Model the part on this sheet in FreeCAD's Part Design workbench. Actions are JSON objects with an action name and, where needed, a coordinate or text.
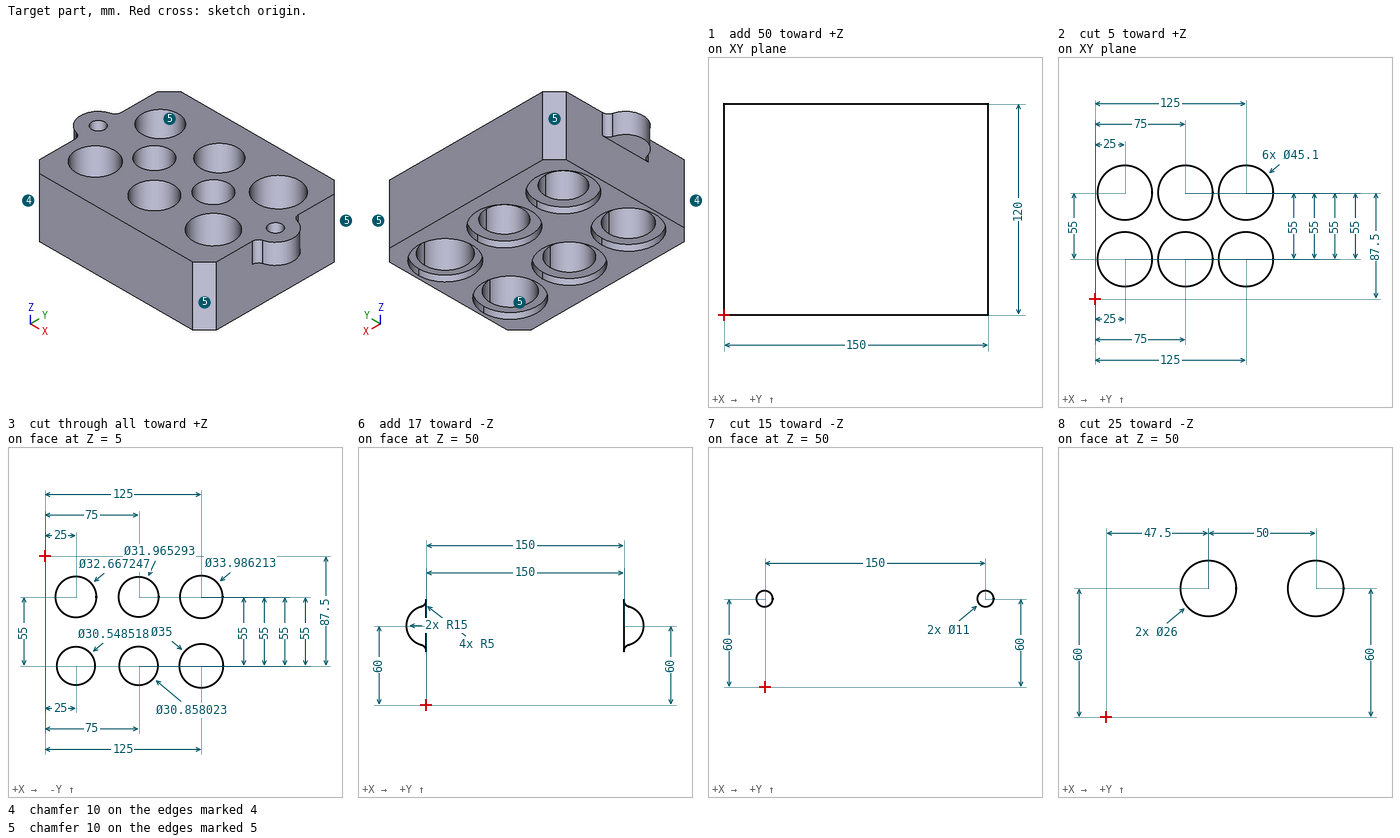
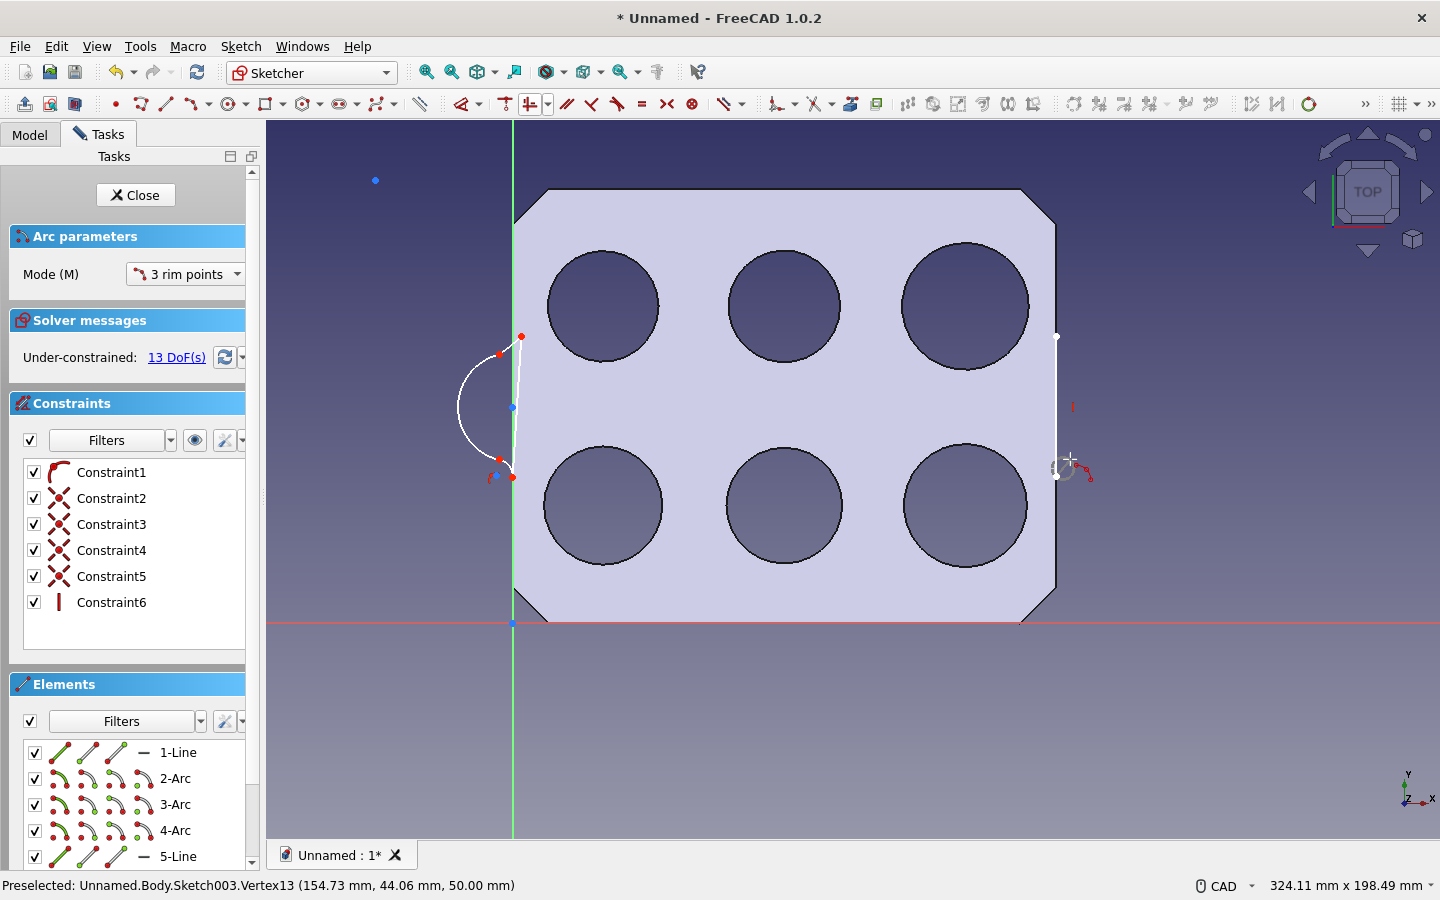
{"action": "scroll", "coordinate": [1060, 465], "scroll_direction": "up", "scroll_amount": 8}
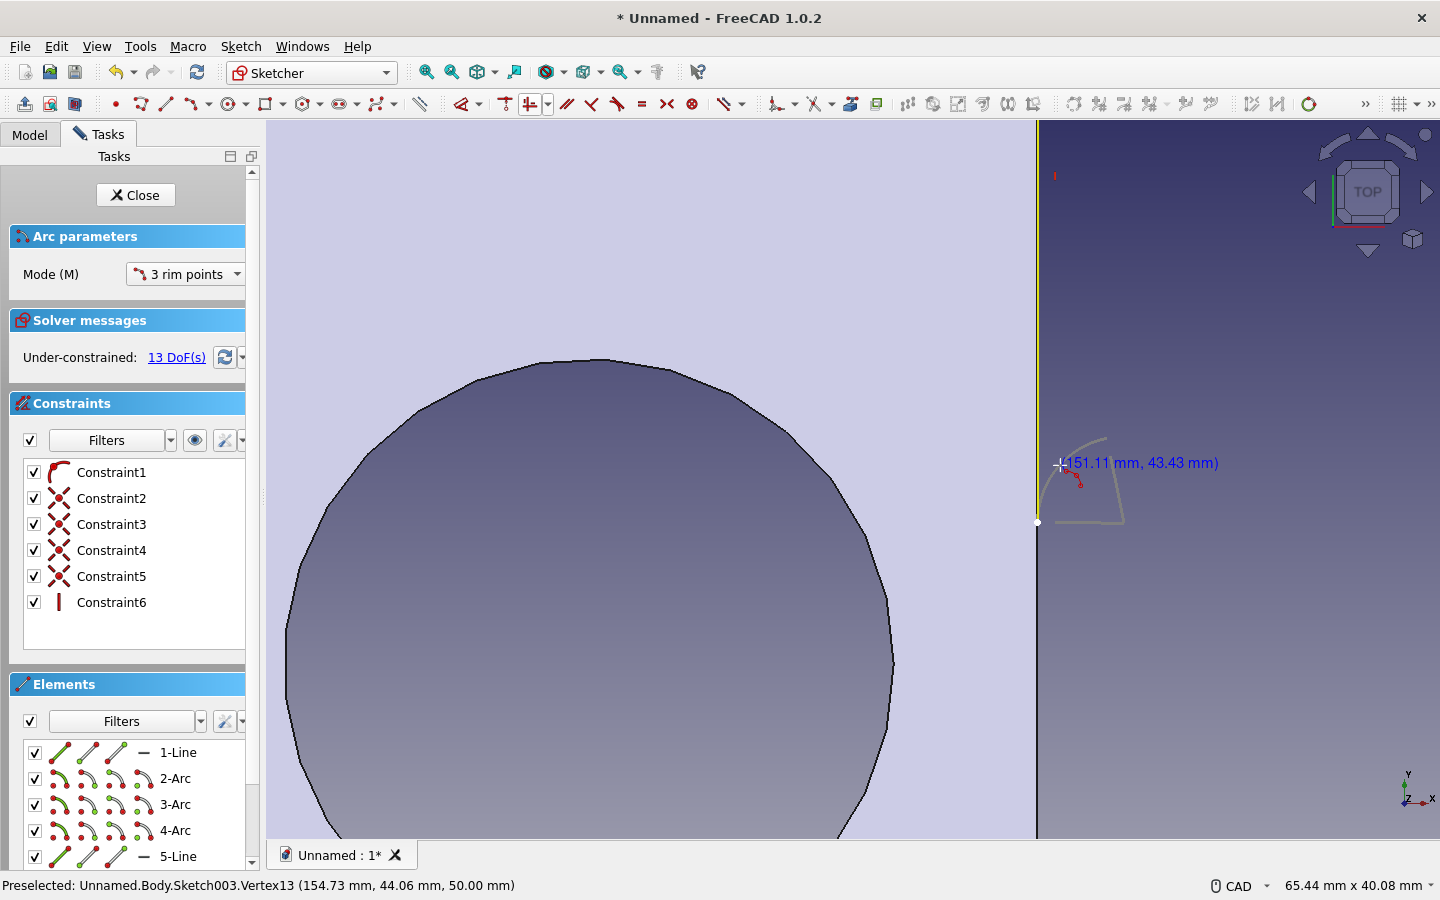
{"action": "left_click", "coordinate": [1056, 463]}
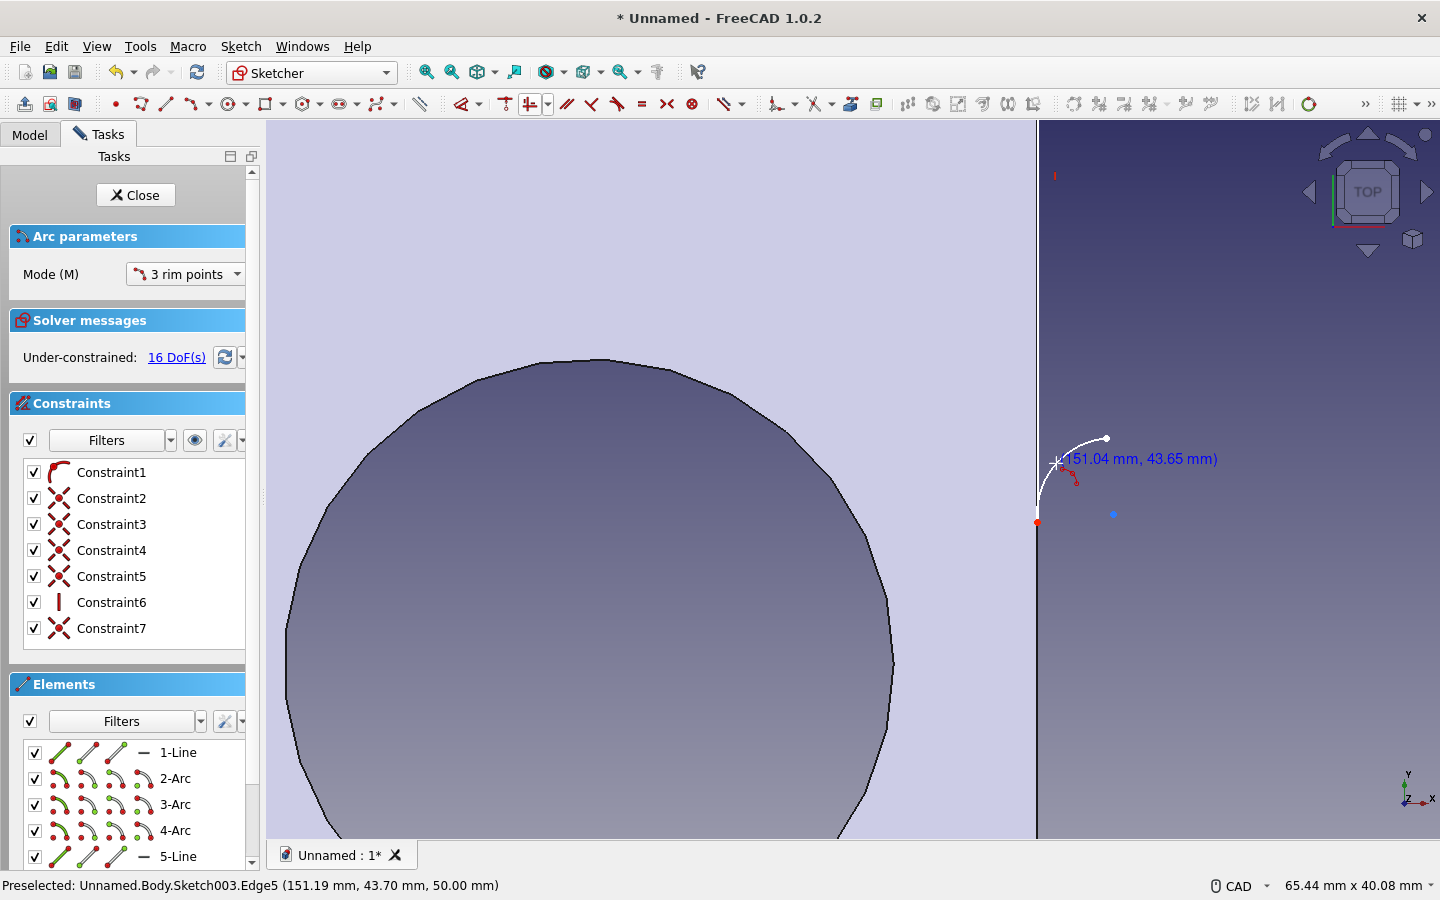
{"action": "scroll", "coordinate": [1061, 465], "scroll_direction": "down", "scroll_amount": 8}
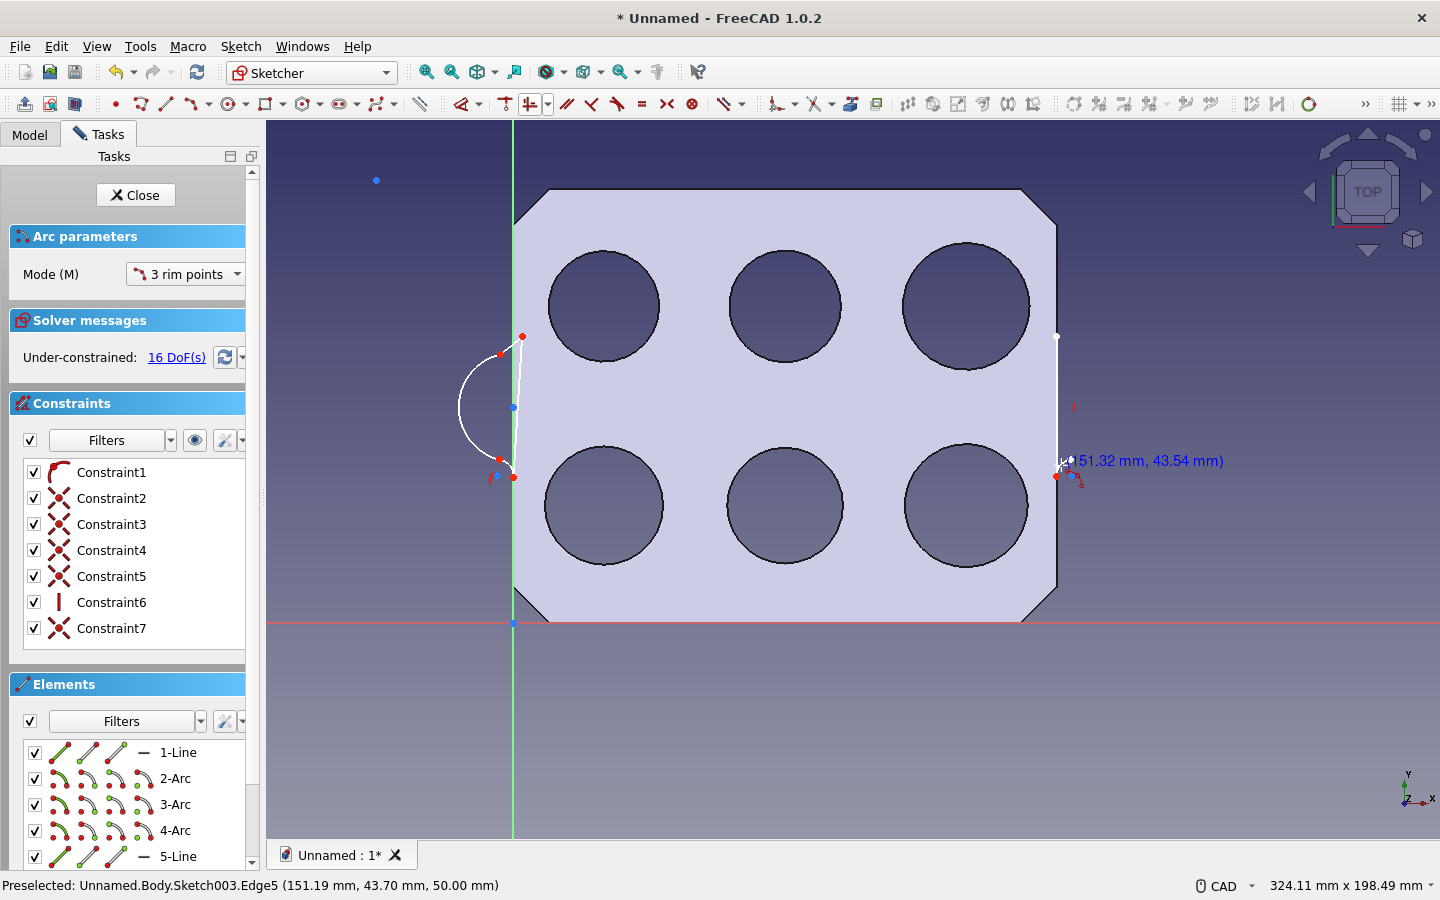
{"action": "left_click", "coordinate": [1071, 460]}
{"action": "left_click", "coordinate": [1070, 353]}
{"action": "left_click", "coordinate": [1111, 406]}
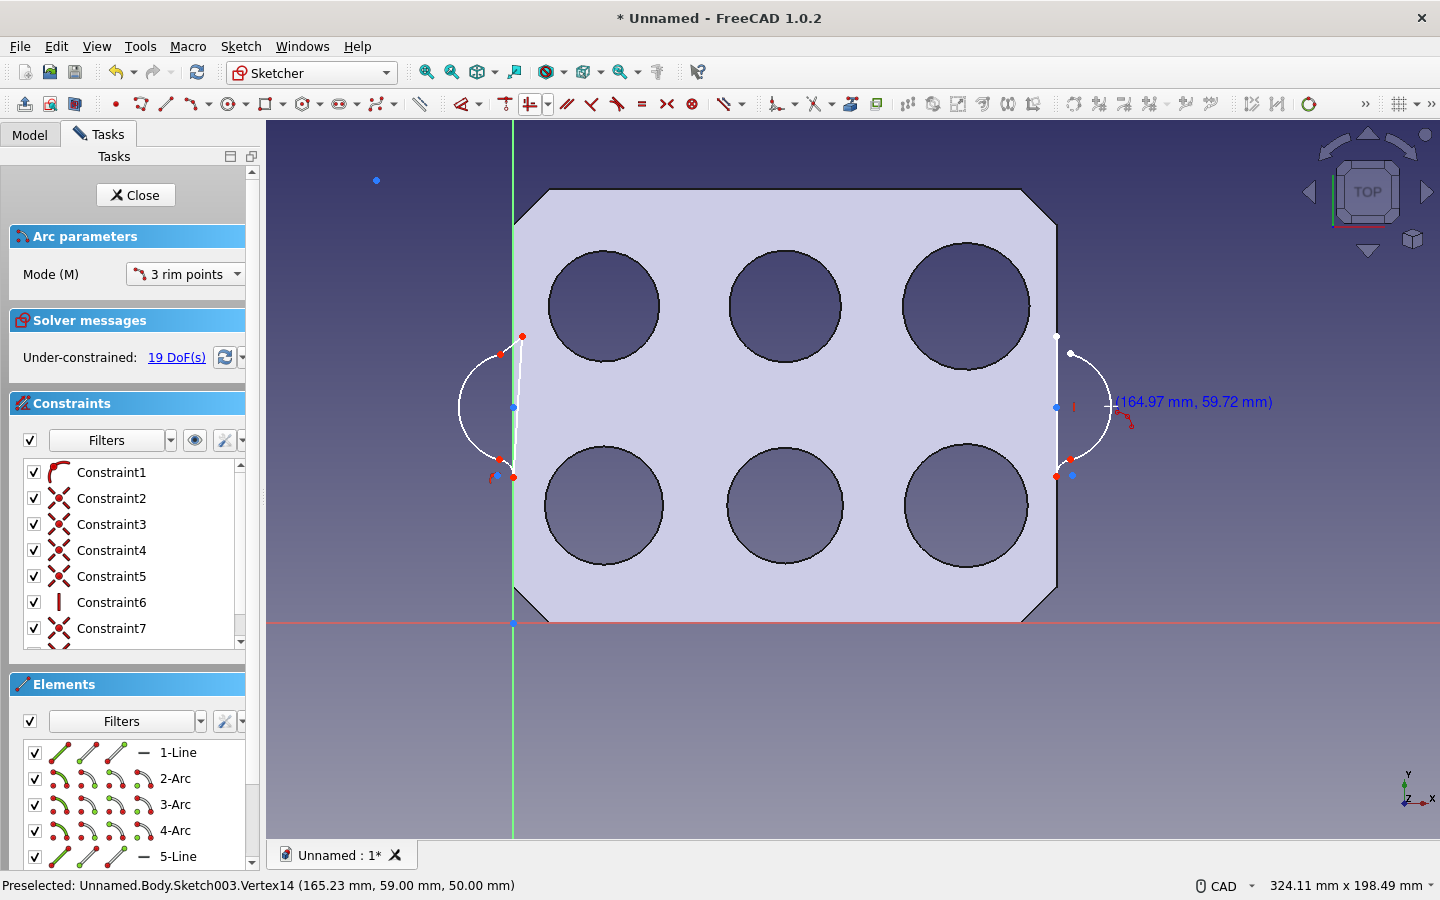
{"action": "left_click", "coordinate": [1070, 354]}
{"action": "left_click", "coordinate": [1057, 337]}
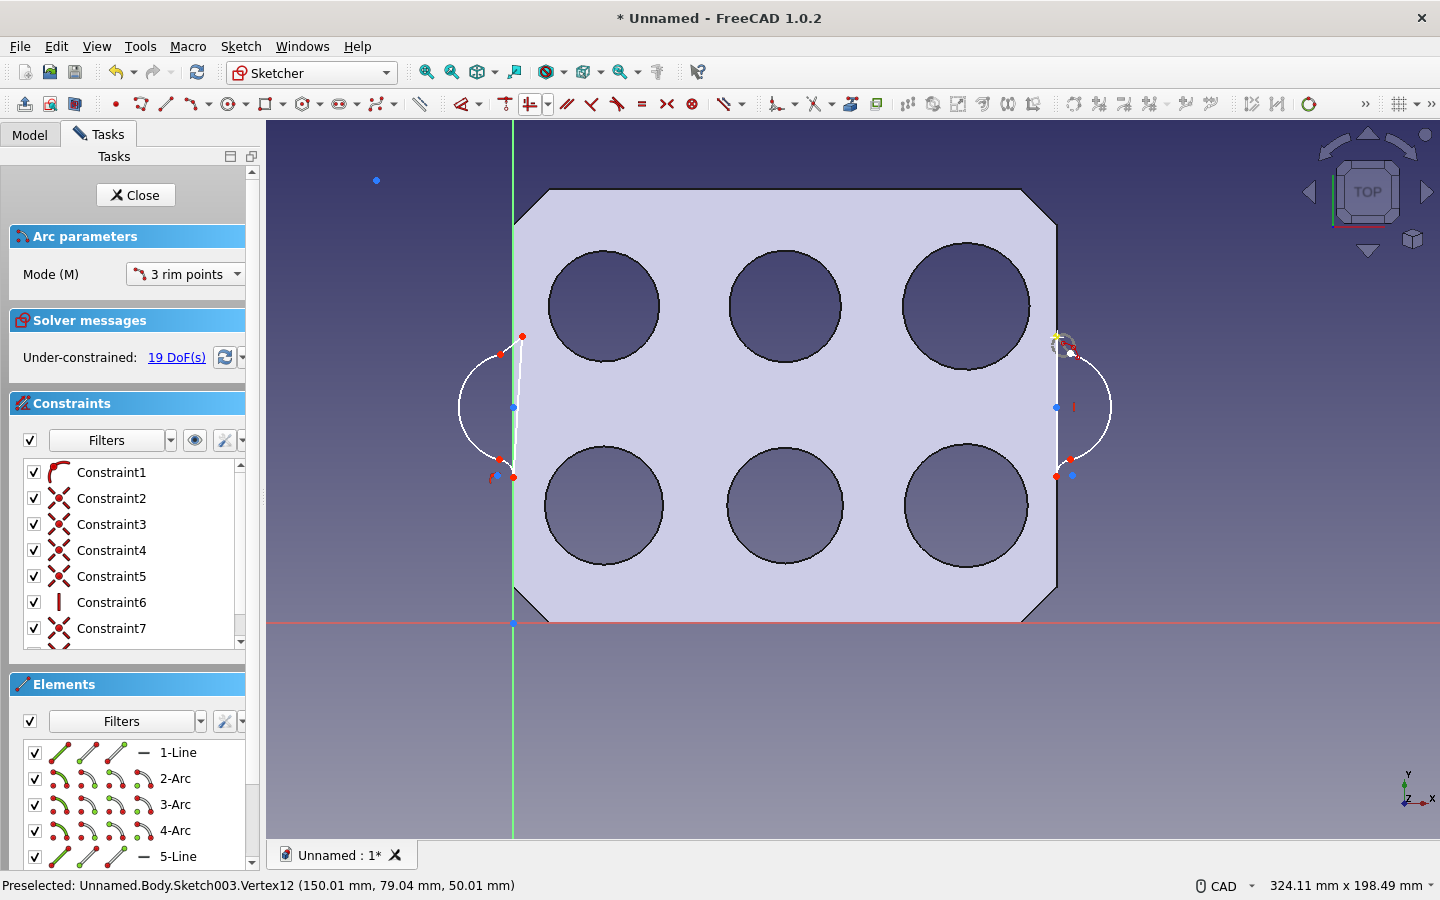
{"action": "scroll", "coordinate": [1061, 347], "scroll_direction": "up", "scroll_amount": 8}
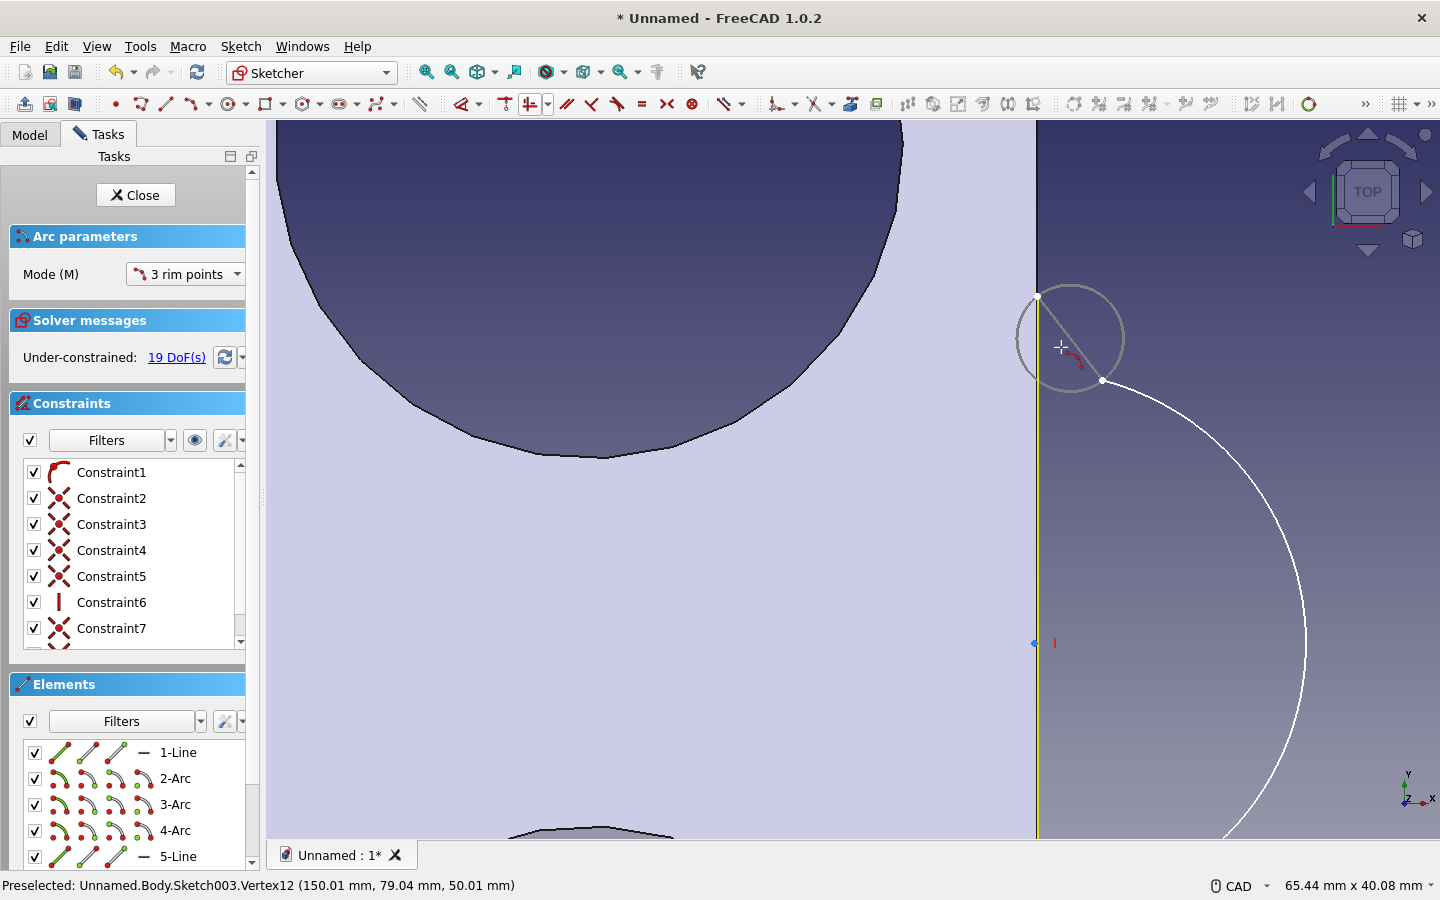
{"action": "left_click", "coordinate": [1056, 345]}
{"action": "key", "text": "Escape"}